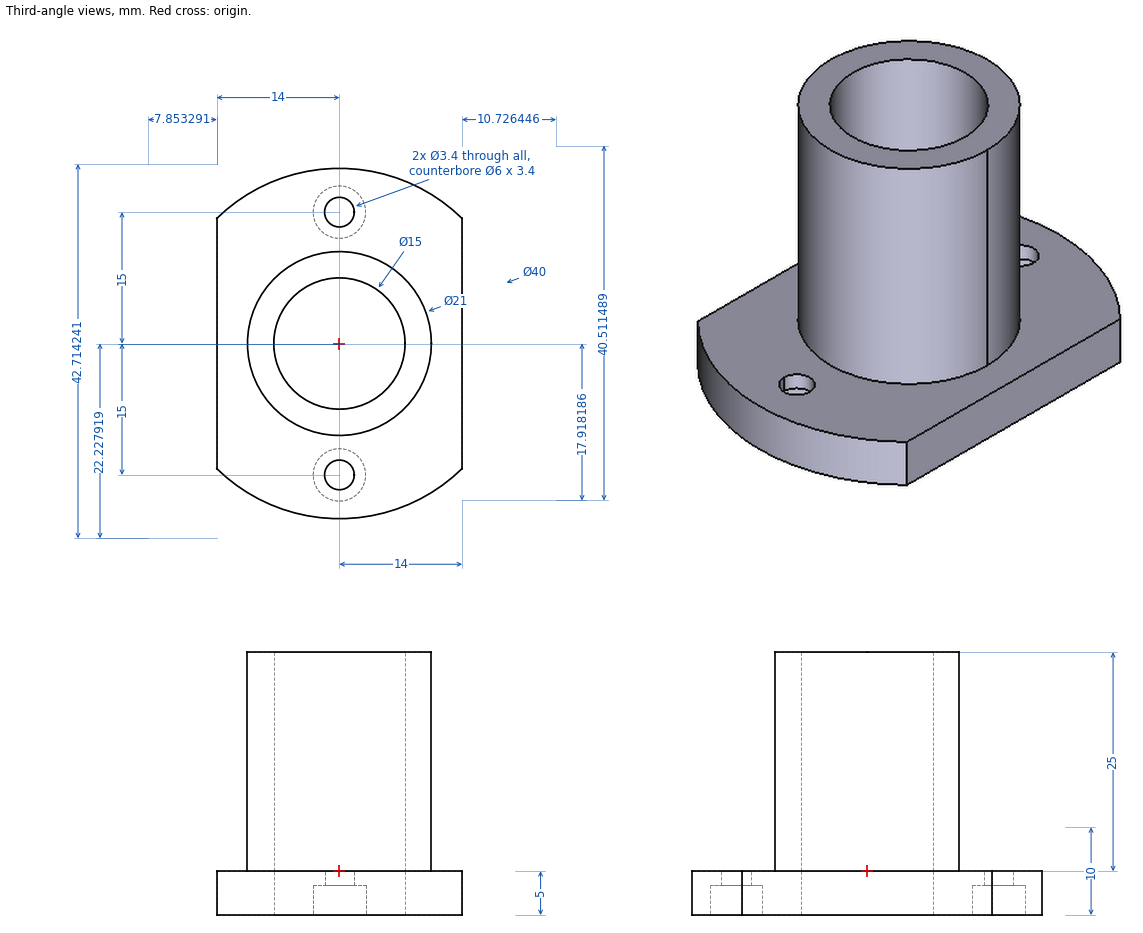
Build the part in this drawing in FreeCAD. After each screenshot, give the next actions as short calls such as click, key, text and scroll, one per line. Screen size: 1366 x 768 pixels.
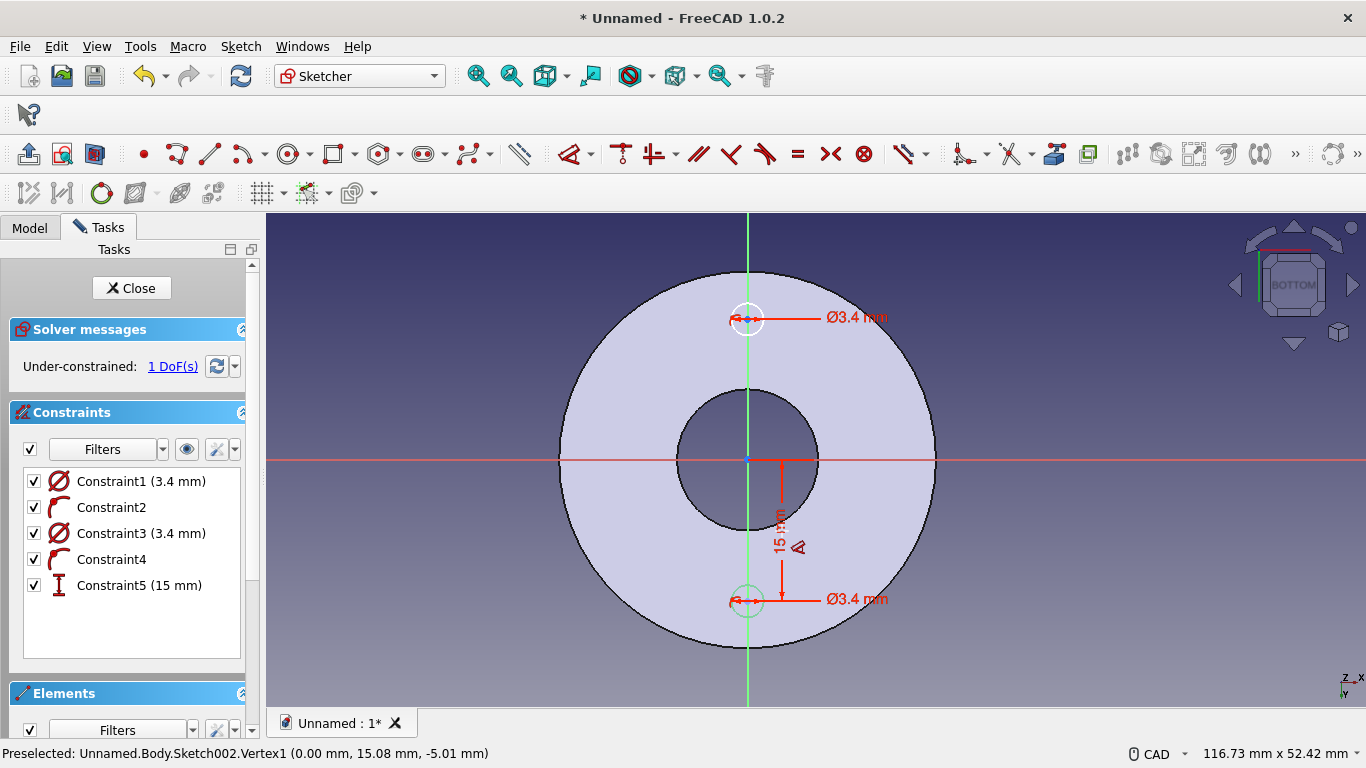
click(748, 319)
click(782, 390)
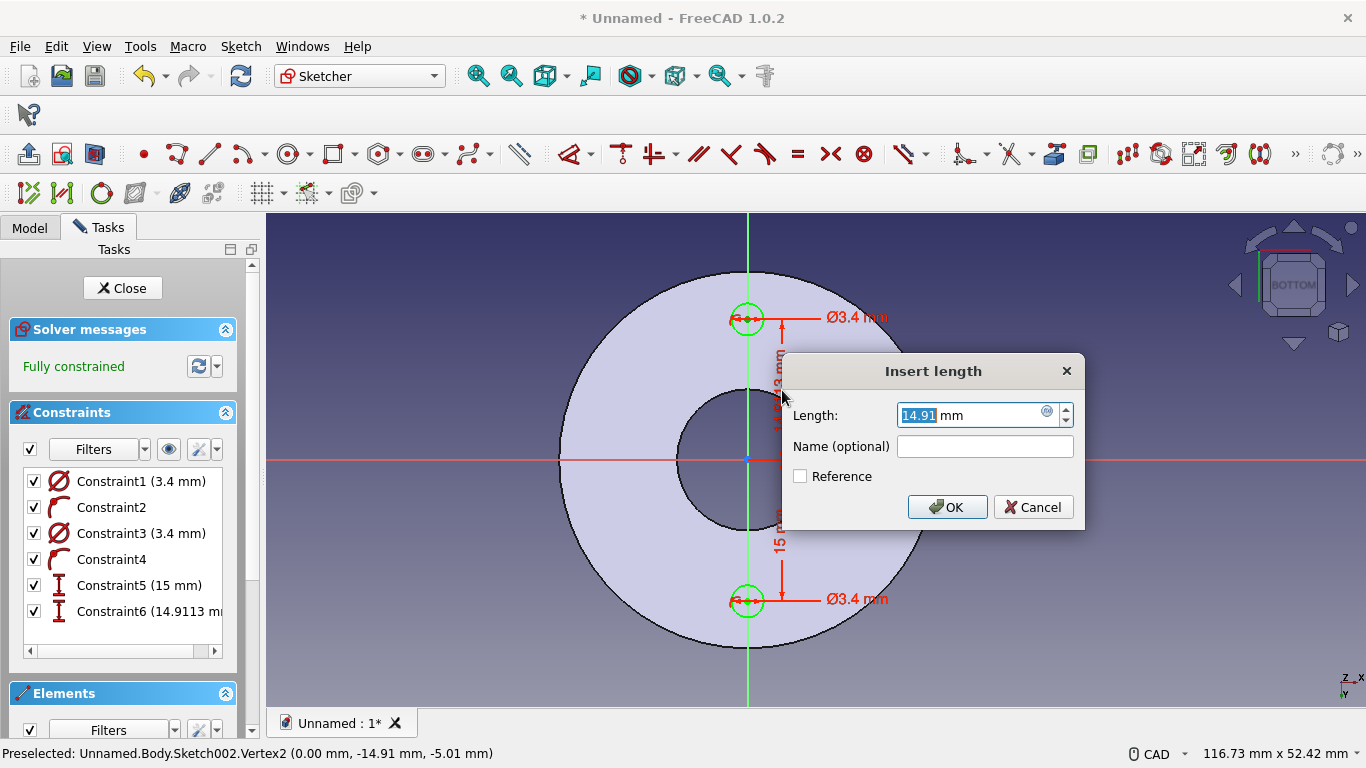
text(15)
key(Return)
key(Escape)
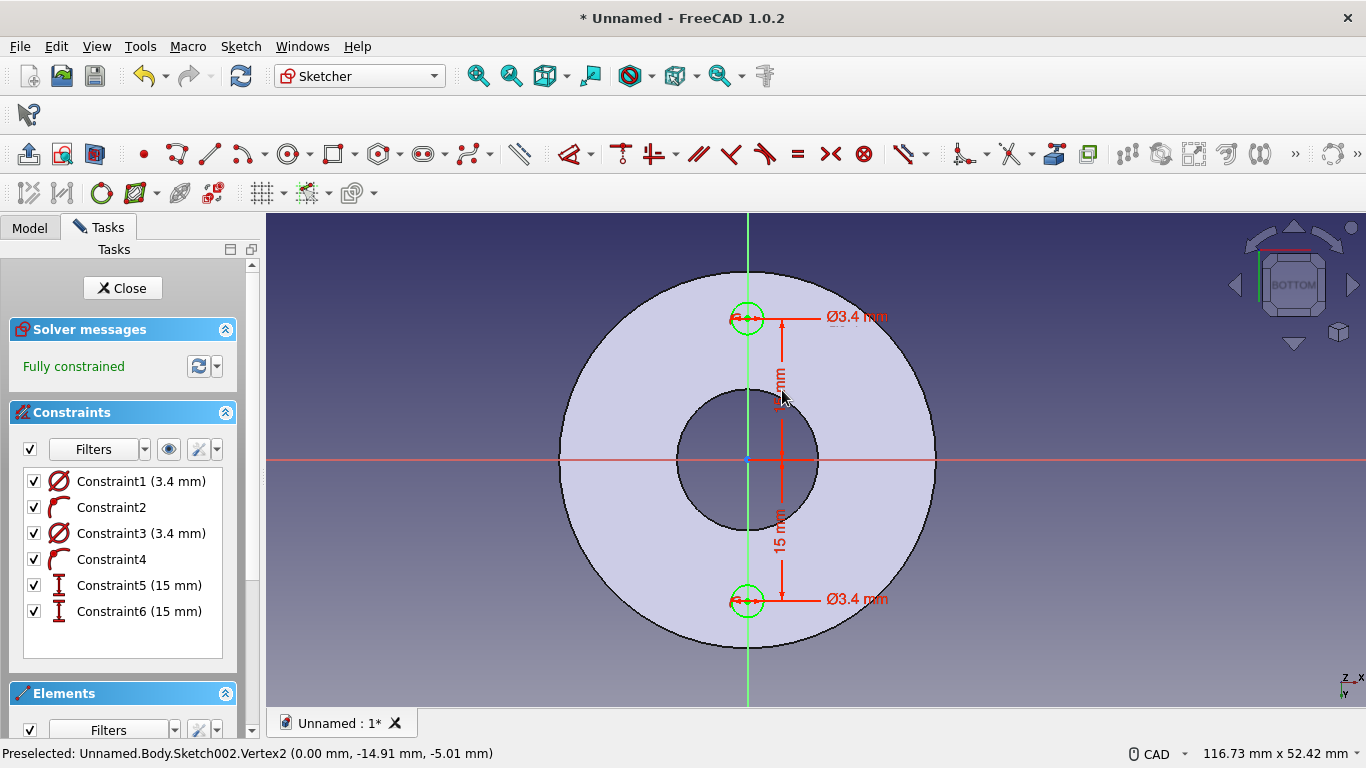
click(123, 288)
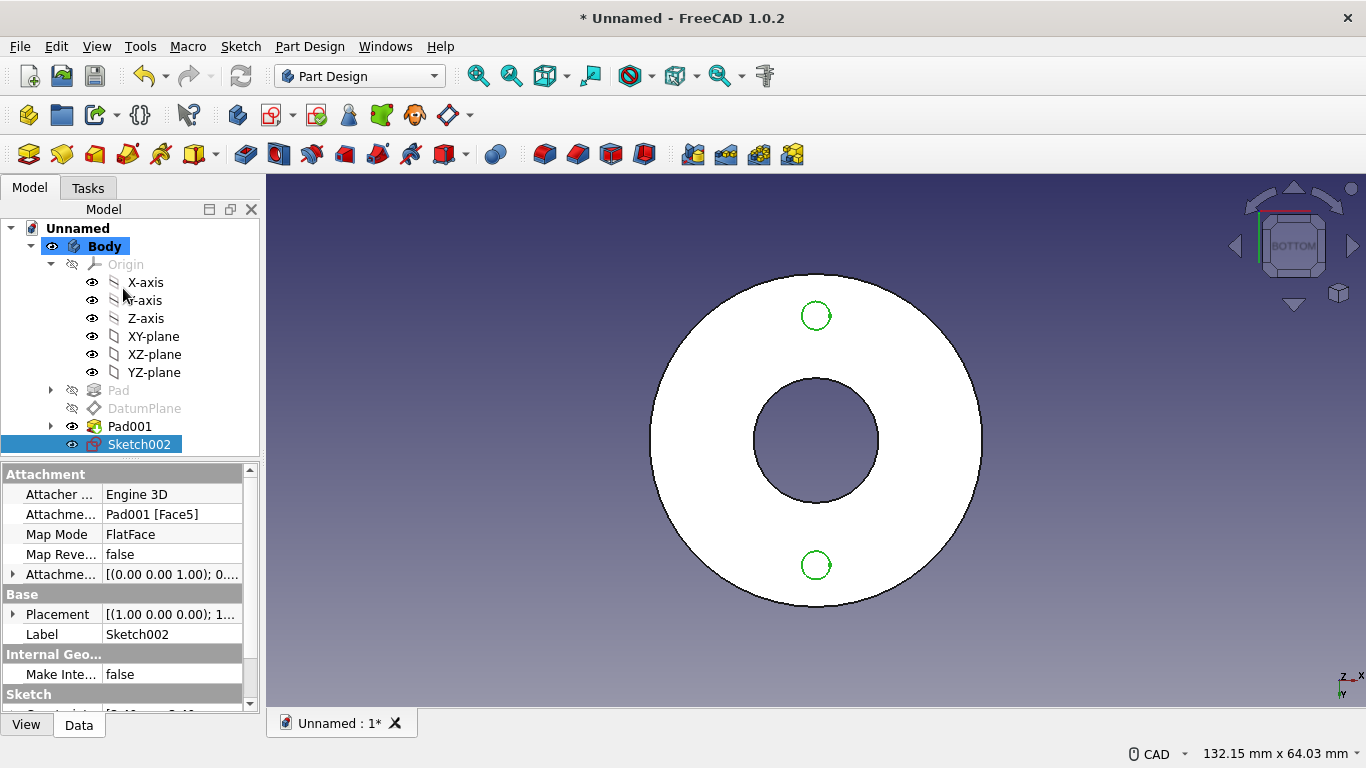
click(279, 154)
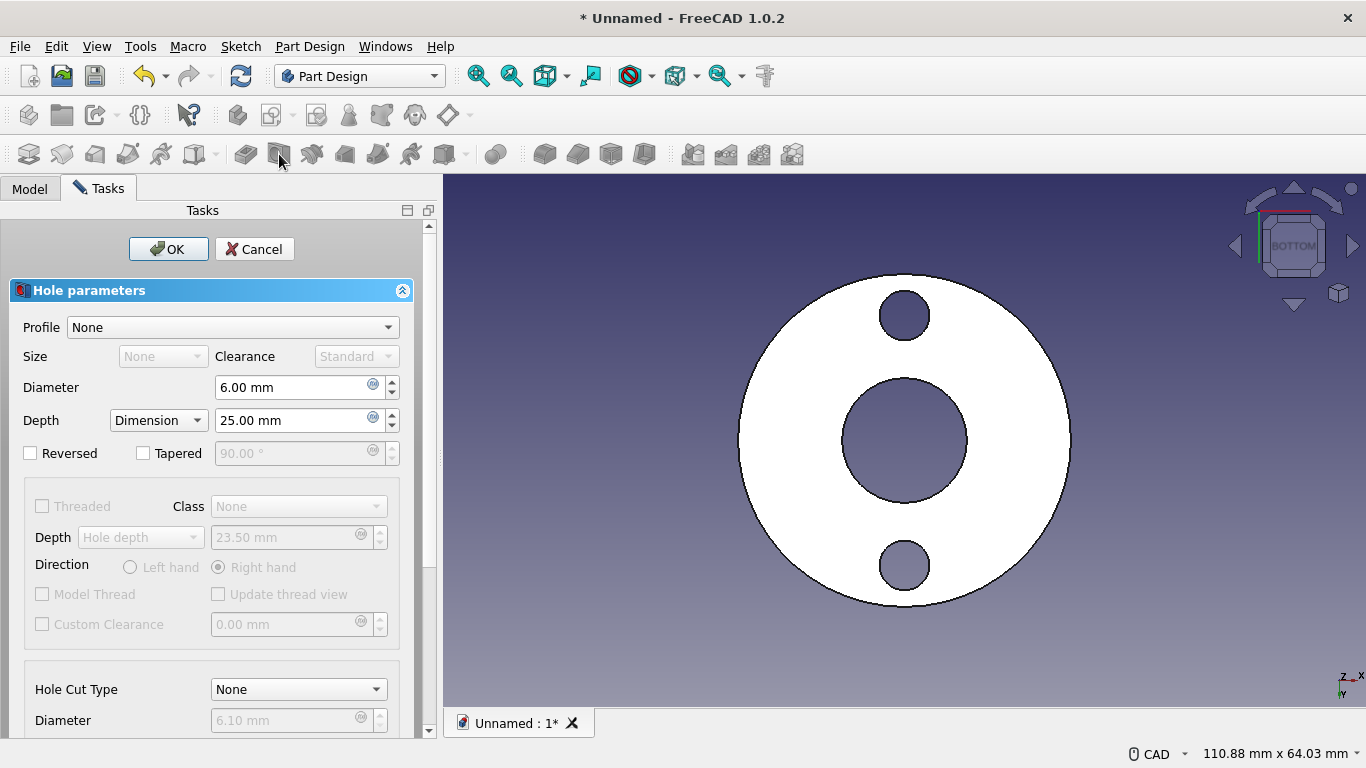
triple_click(300, 388)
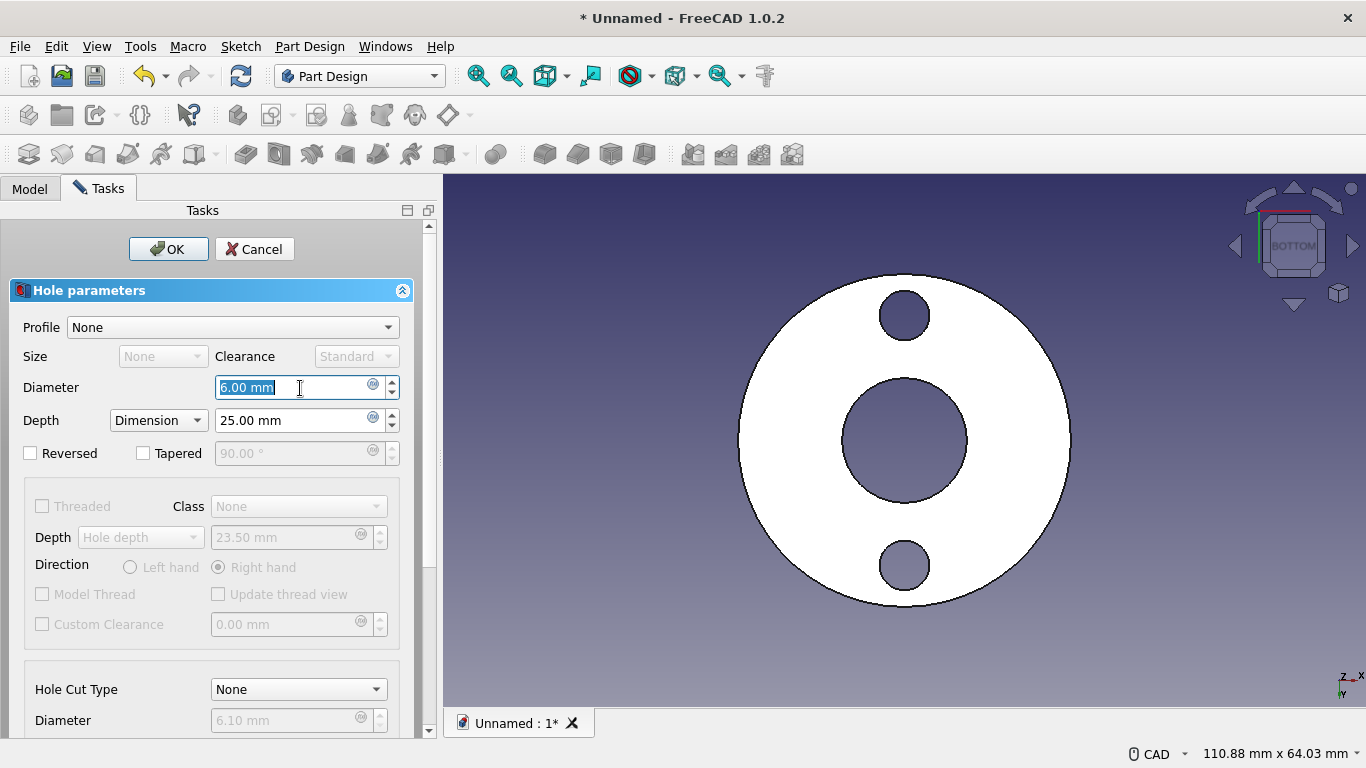
text(3.4)
key(Tab)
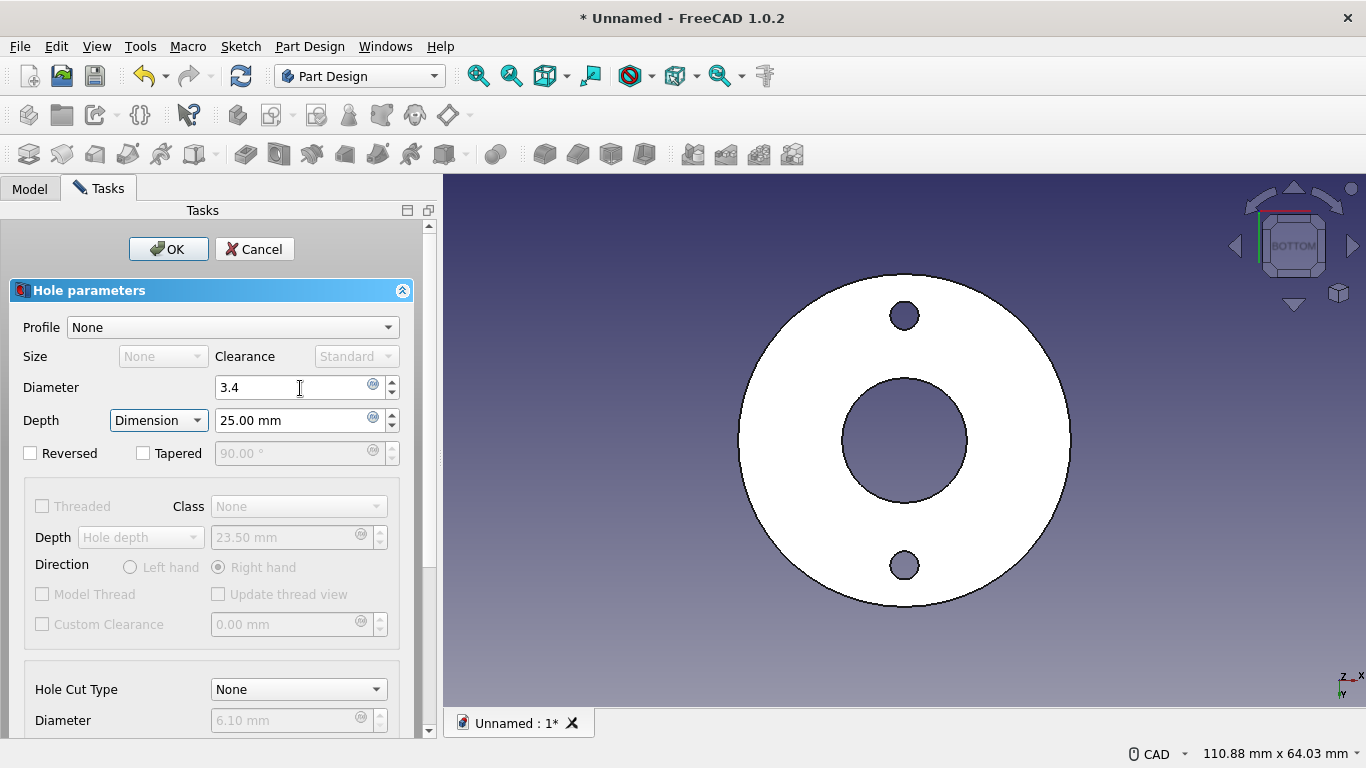
click(160, 420)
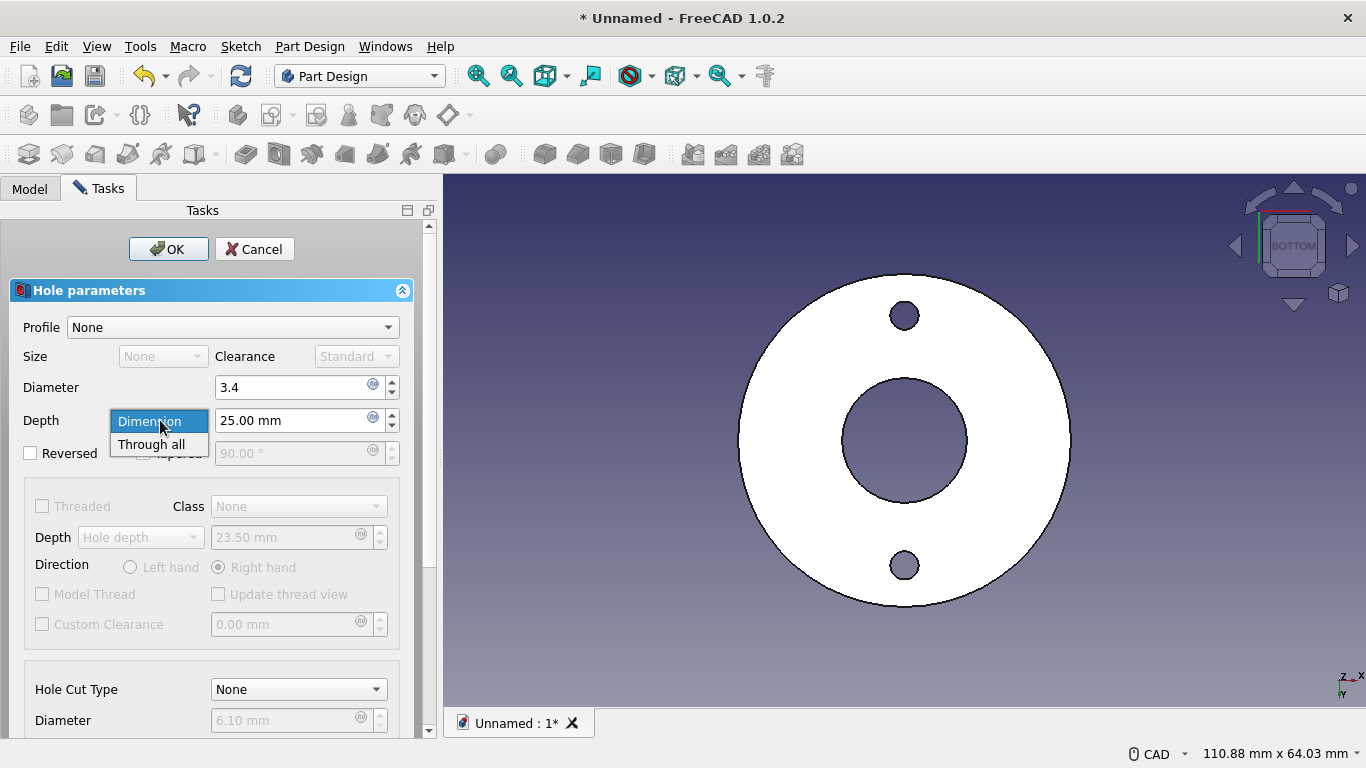
click(158, 444)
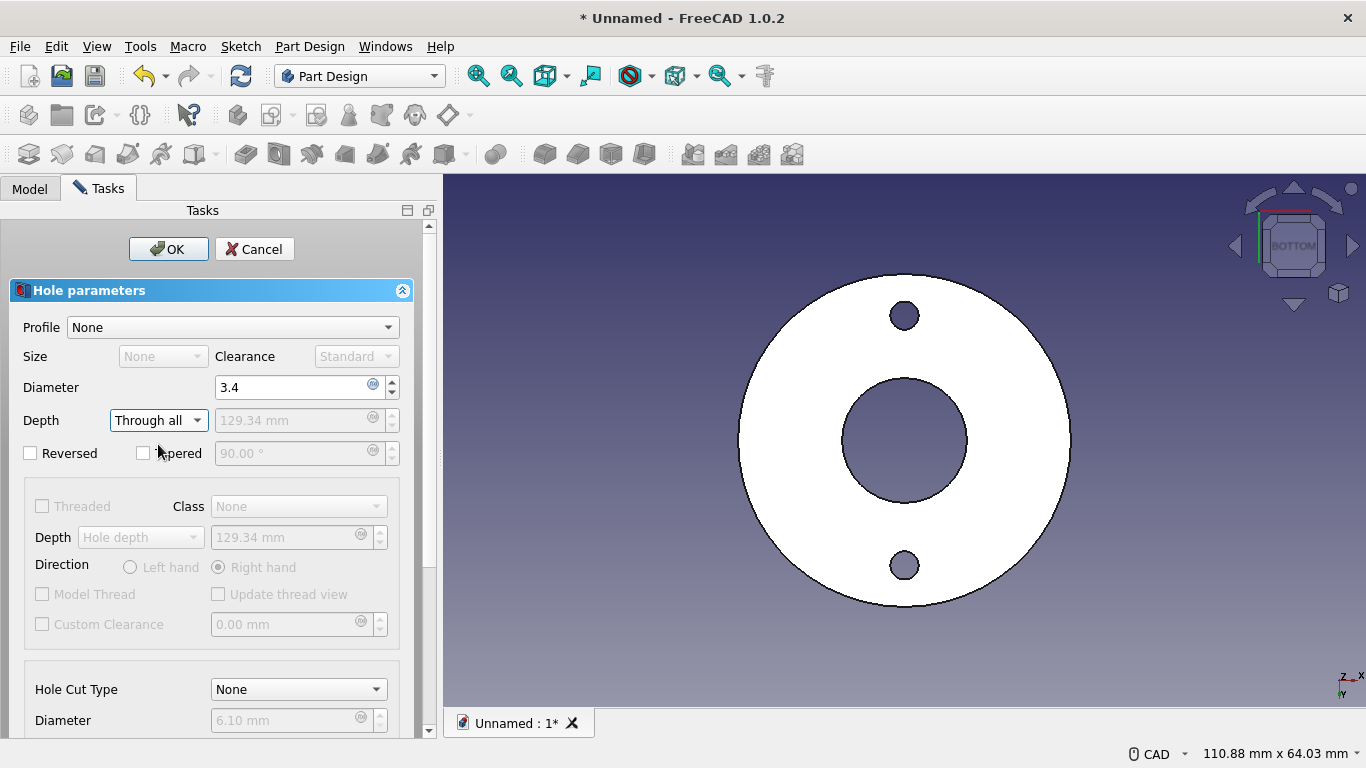
click(300, 690)